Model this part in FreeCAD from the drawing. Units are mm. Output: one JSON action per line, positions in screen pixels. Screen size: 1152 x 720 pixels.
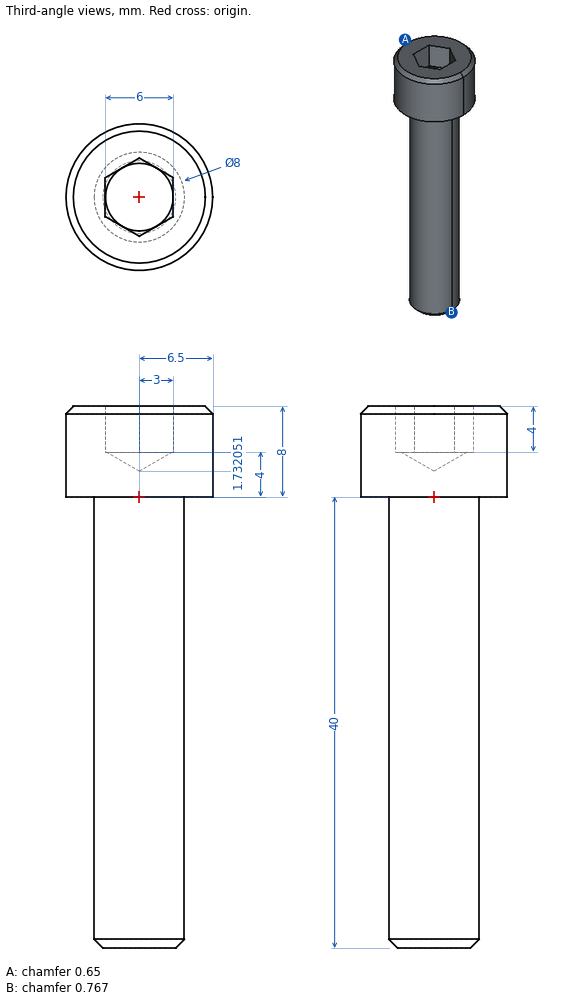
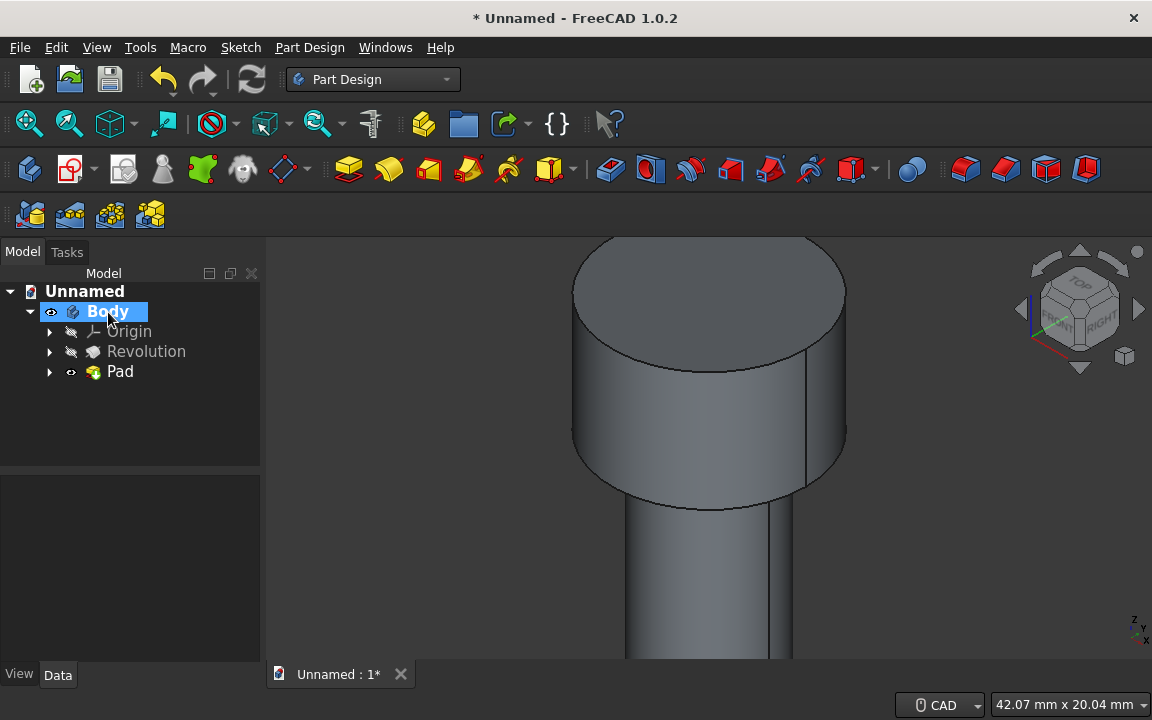
{"action": "left_click", "coordinate": [30, 124]}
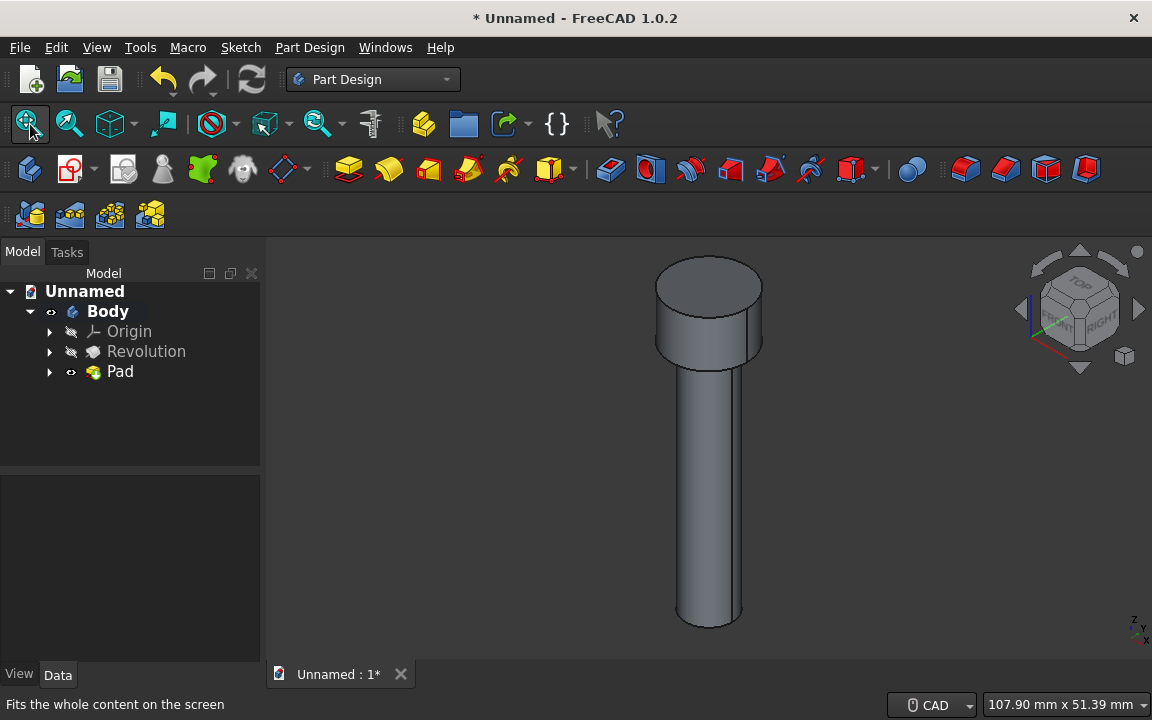
{"action": "left_click", "coordinate": [709, 286]}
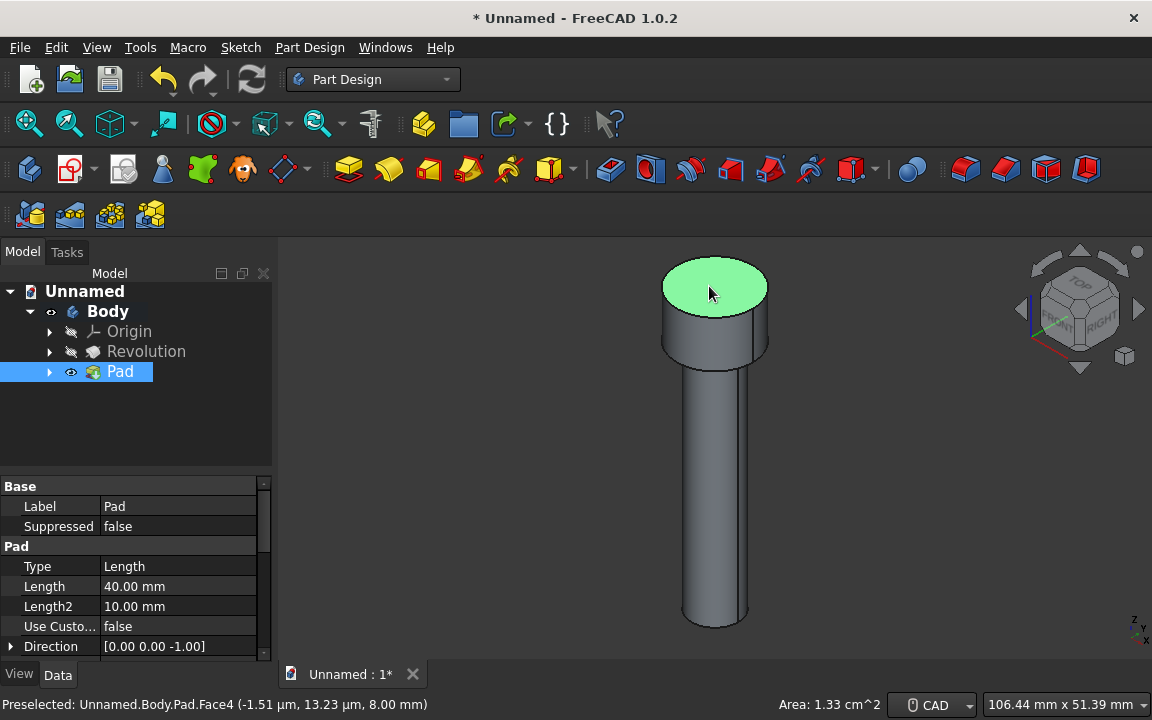
{"action": "left_click", "coordinate": [70, 170]}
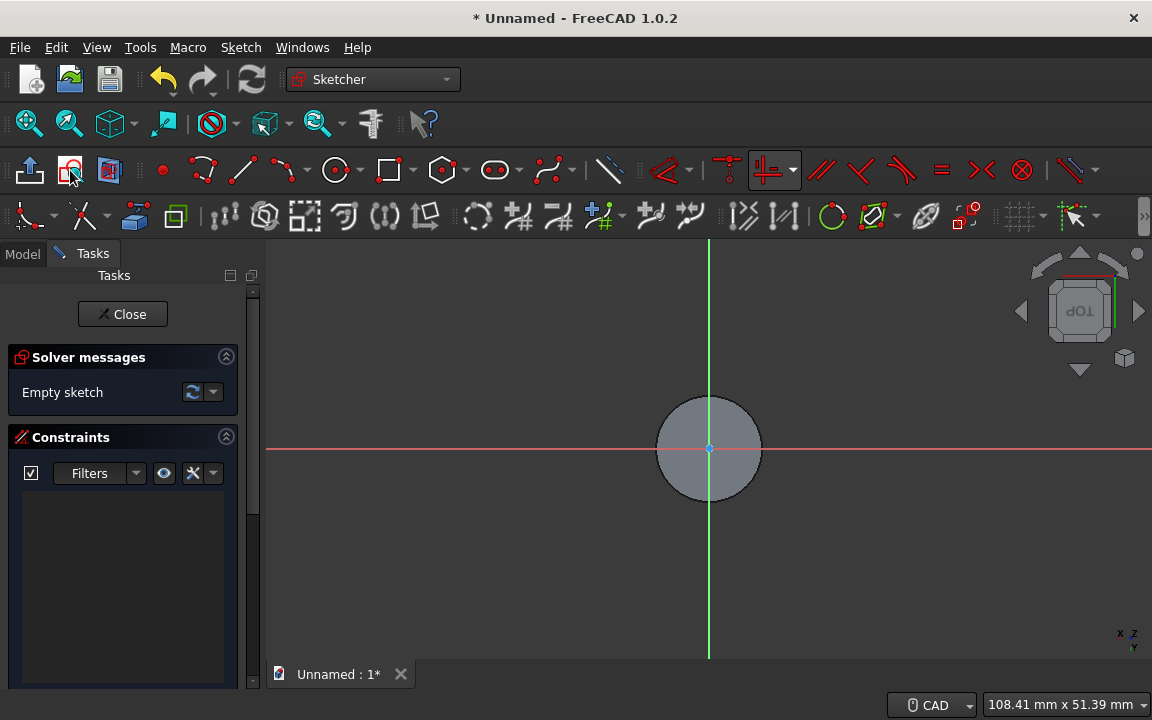
{"action": "scroll", "coordinate": [726, 449], "scroll_direction": "up", "scroll_amount": 8}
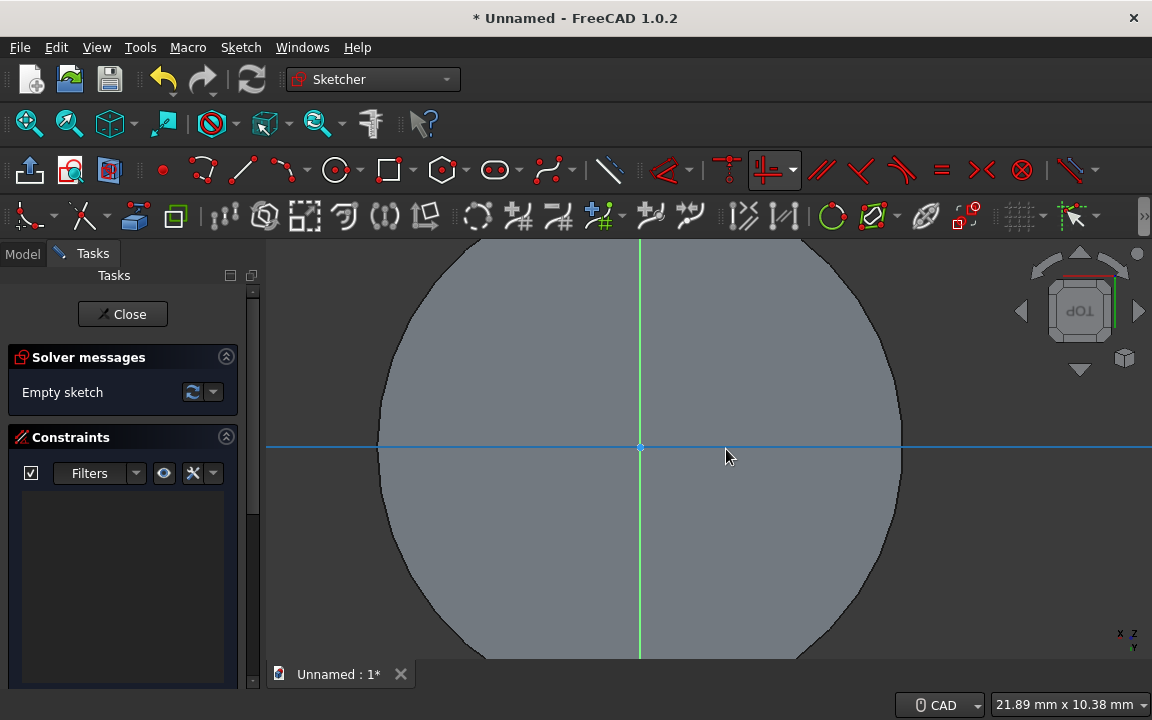
{"action": "left_click", "coordinate": [442, 170]}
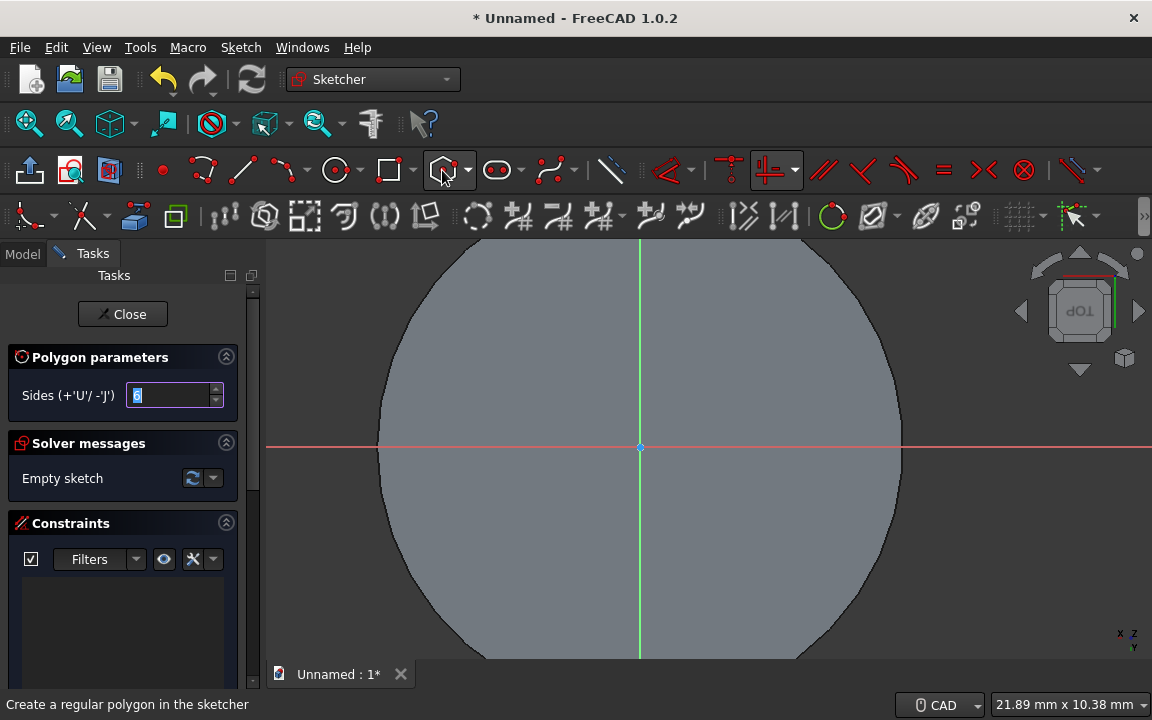
{"action": "left_click", "coordinate": [640, 447]}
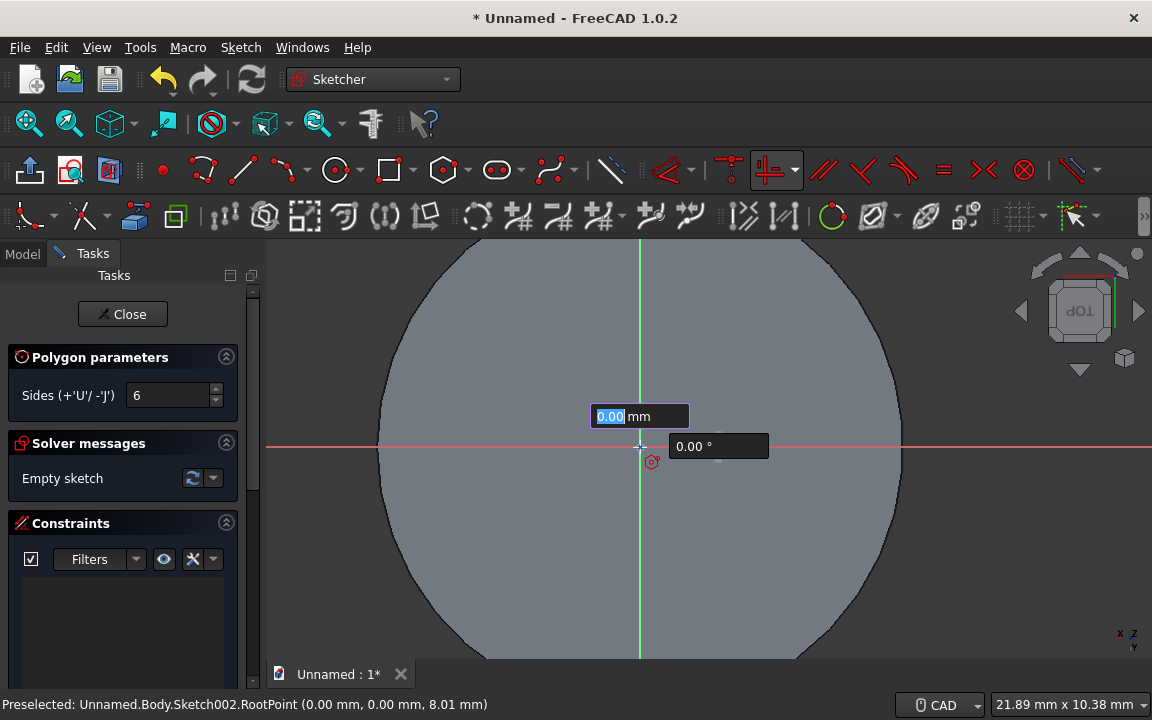
{"action": "left_click", "coordinate": [640, 587]}
{"action": "right_click", "coordinate": [640, 587]}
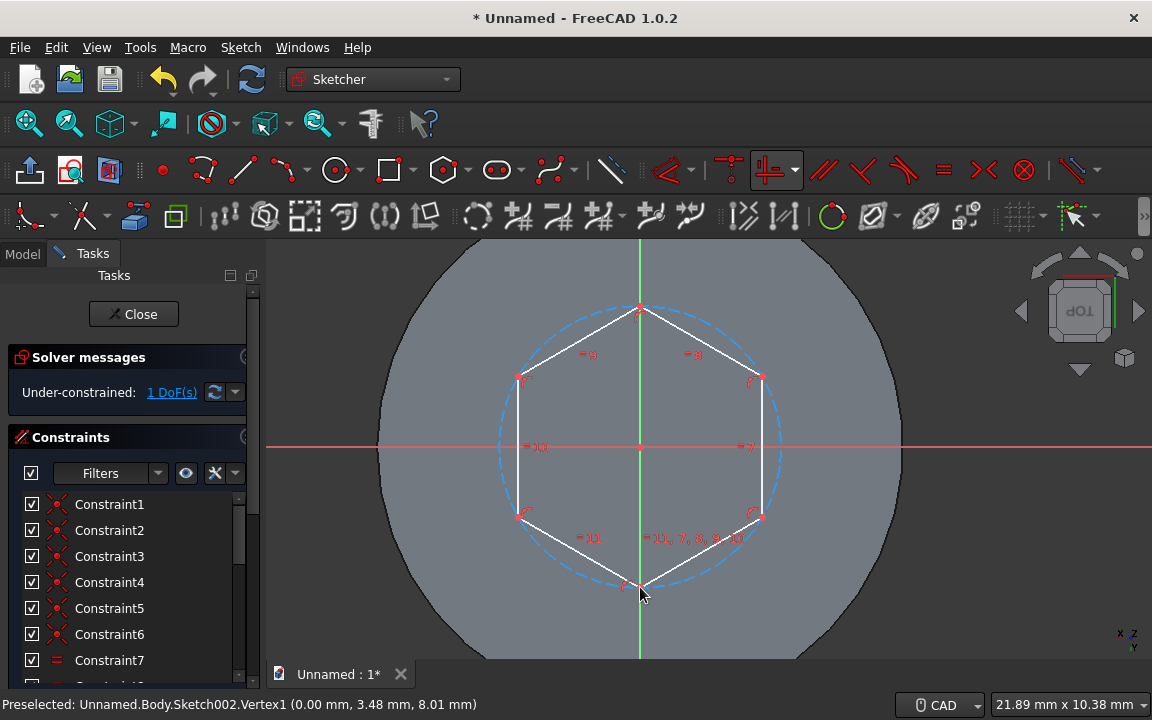
{"action": "left_click", "coordinate": [666, 170]}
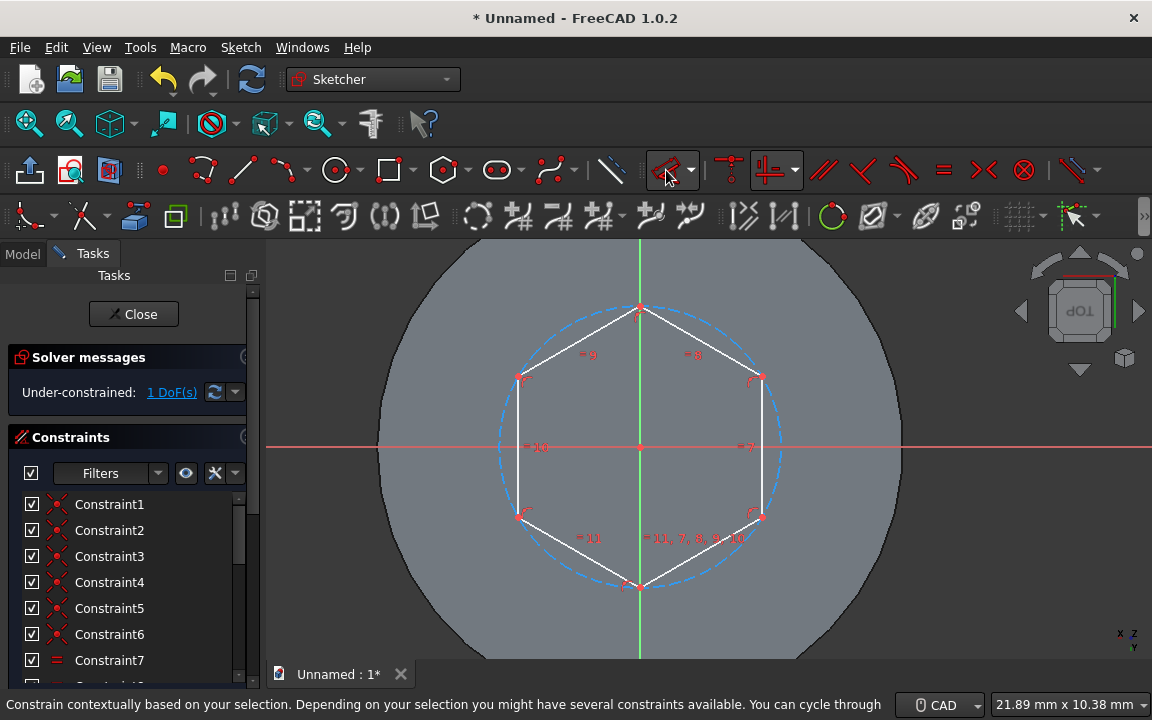
{"action": "left_click", "coordinate": [518, 377]}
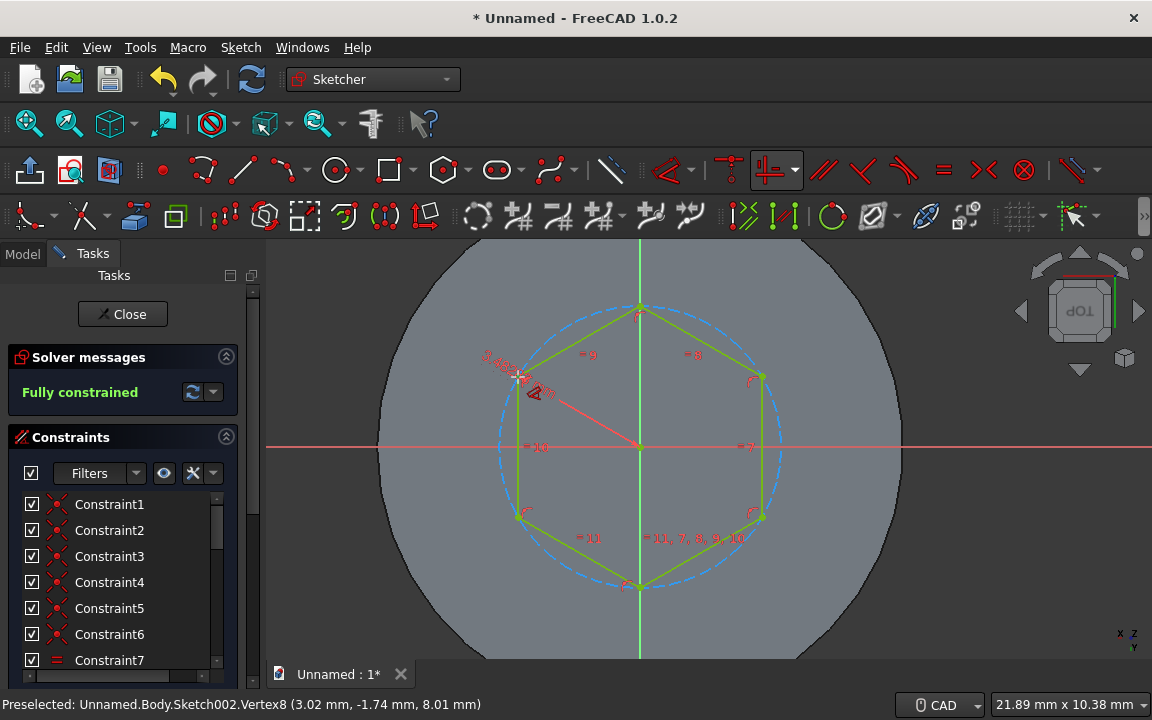
{"action": "left_click", "coordinate": [762, 518]}
{"action": "left_click", "coordinate": [555, 319]}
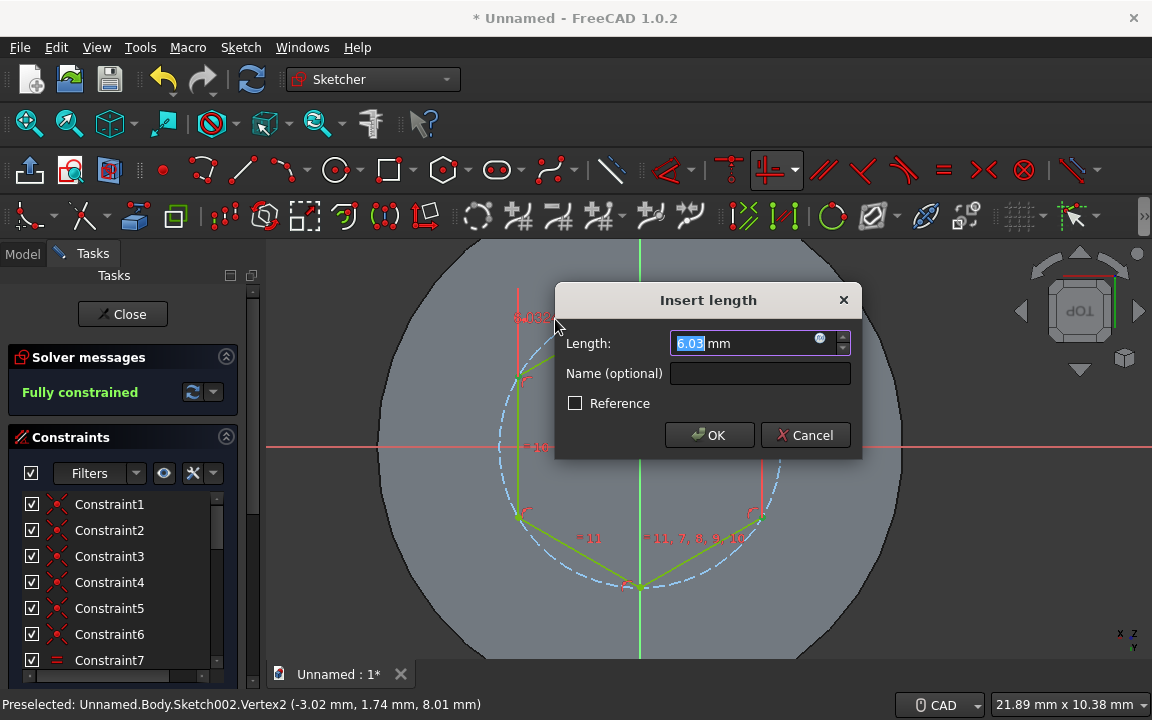
{"action": "type", "text": "6"}
{"action": "key", "text": "Return"}
{"action": "key", "text": "Escape"}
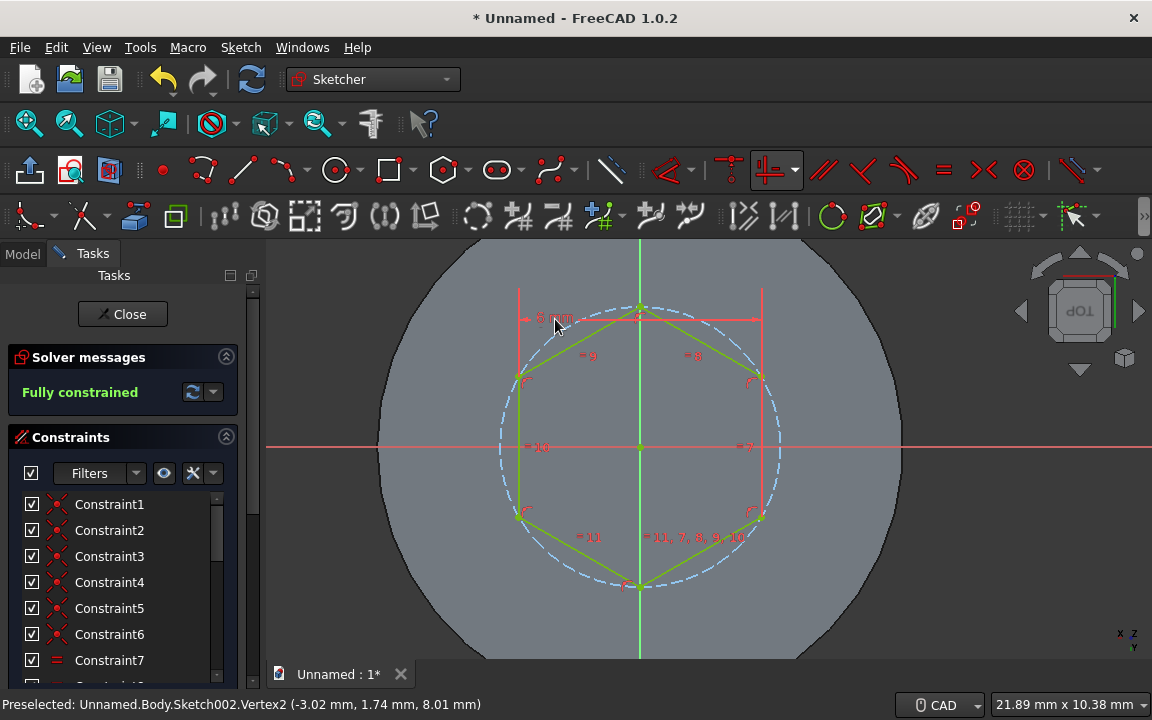
{"action": "left_click", "coordinate": [123, 314]}